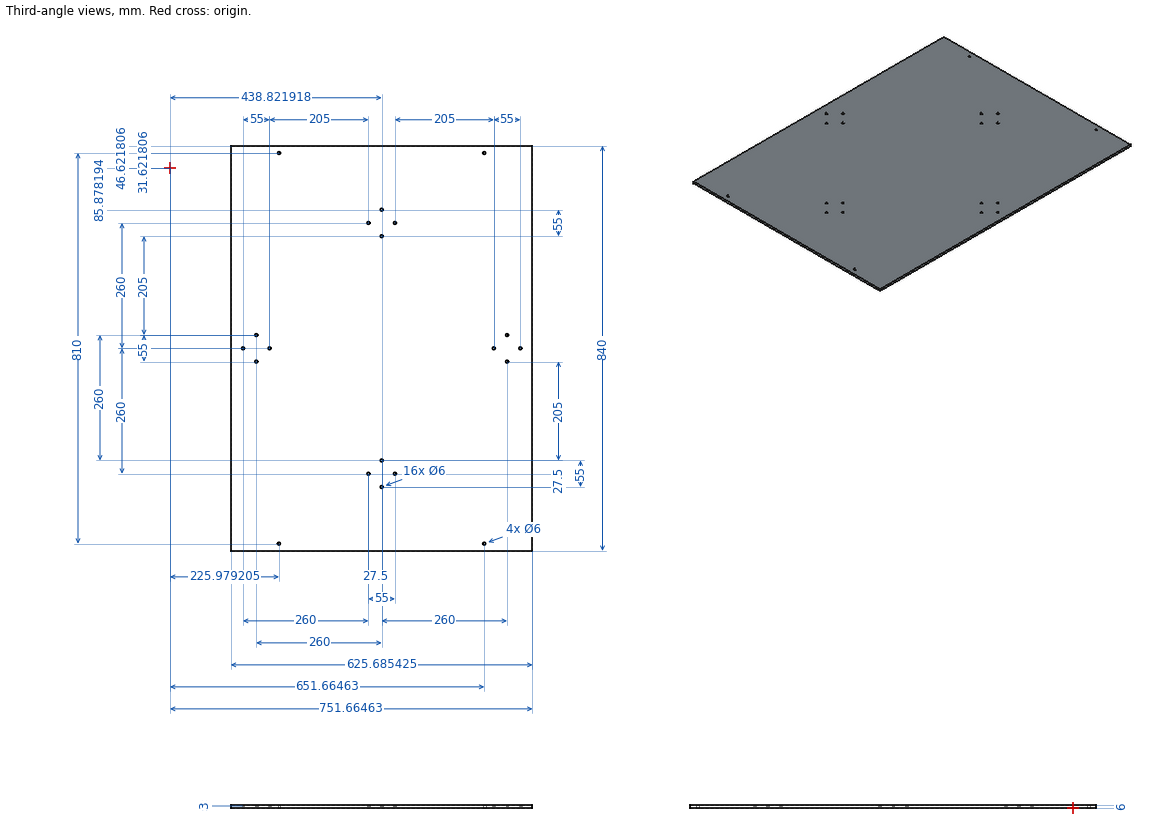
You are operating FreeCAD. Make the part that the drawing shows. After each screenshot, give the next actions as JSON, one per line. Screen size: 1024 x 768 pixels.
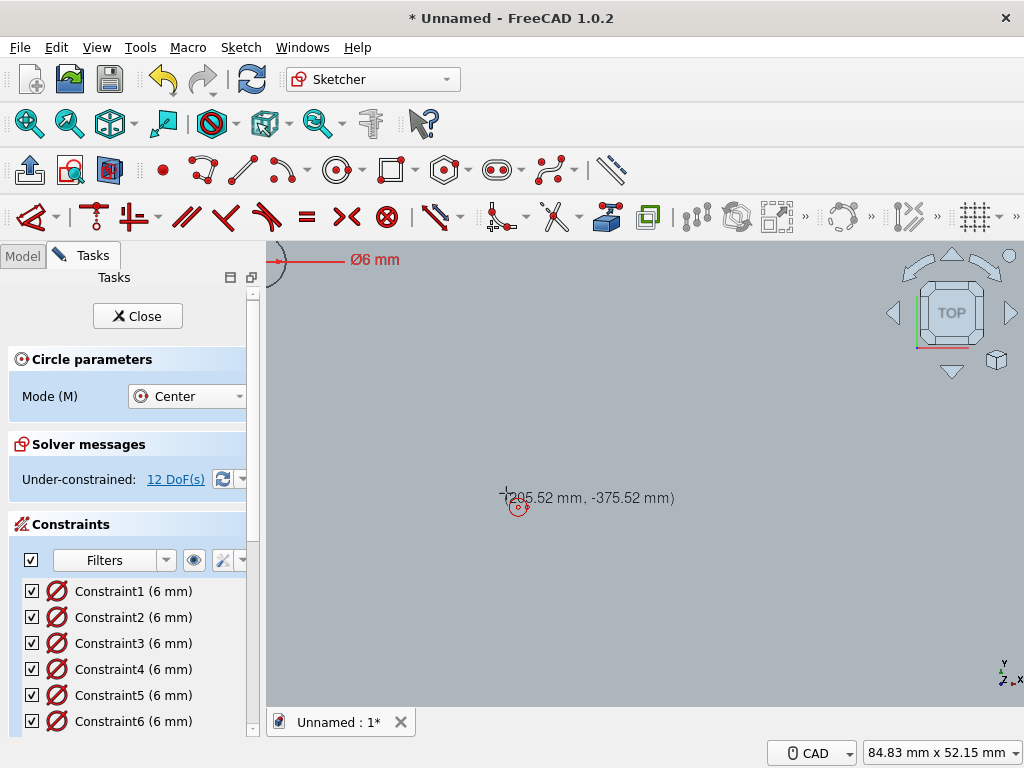
{"action": "scroll", "coordinate": [506, 493], "scroll_direction": "down", "scroll_amount": 15}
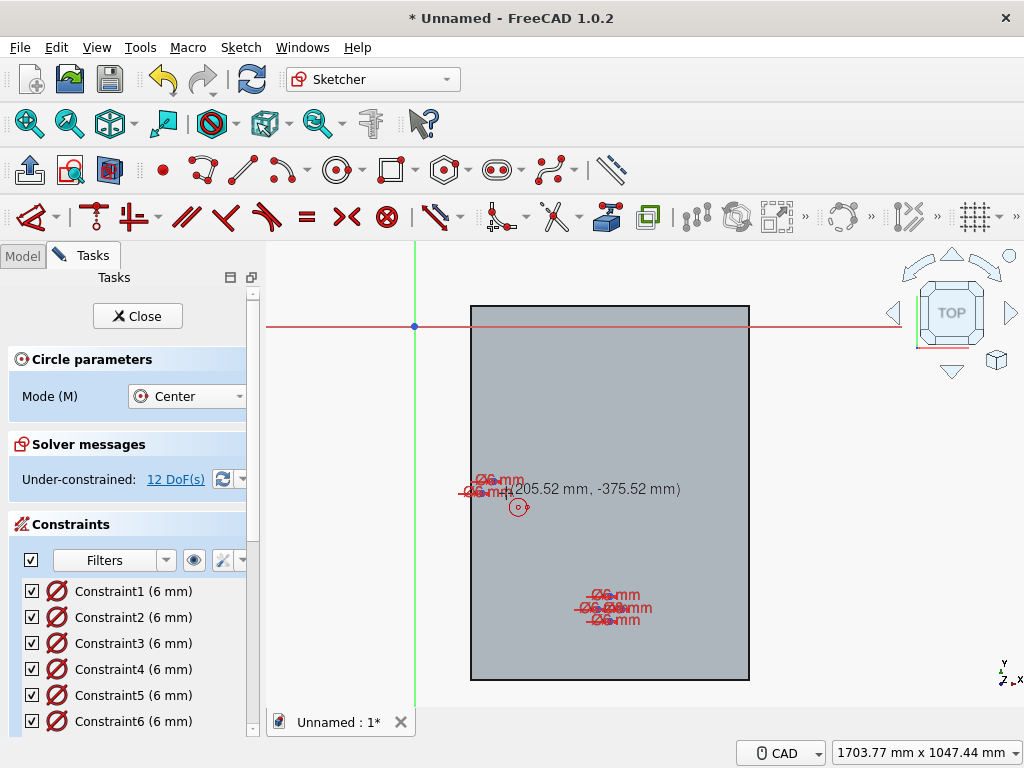
{"action": "left_click", "coordinate": [506, 493]}
{"action": "mouse_move", "coordinate": [507, 492]}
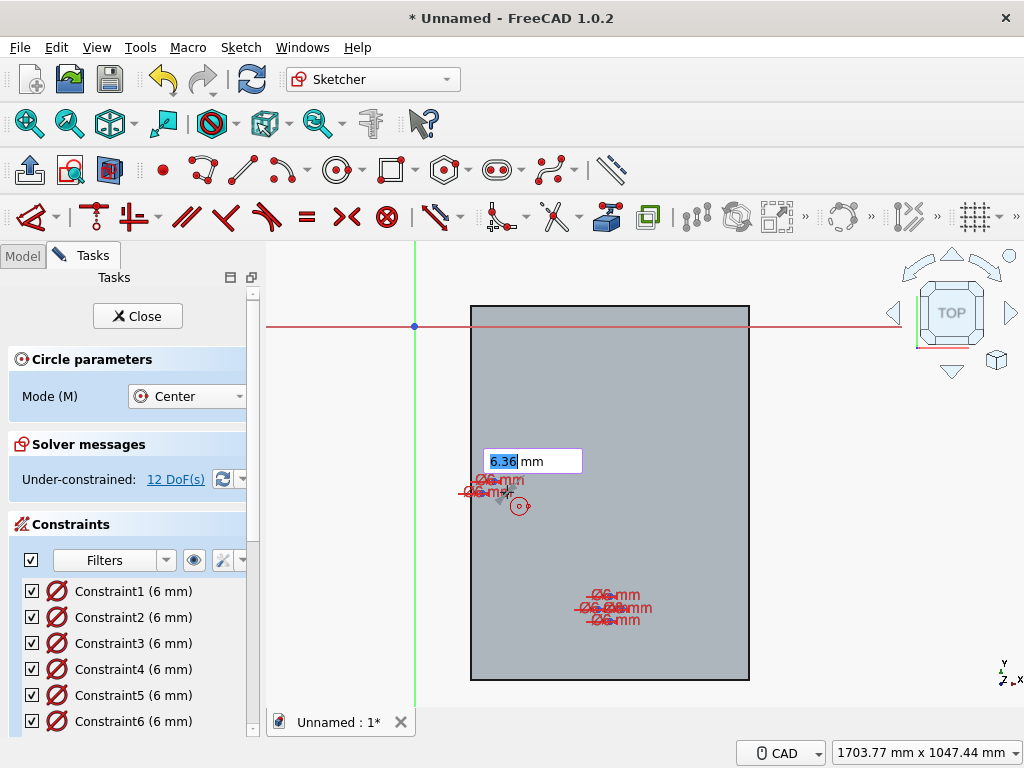
{"action": "type", "text": "6"}
{"action": "key", "text": "Return"}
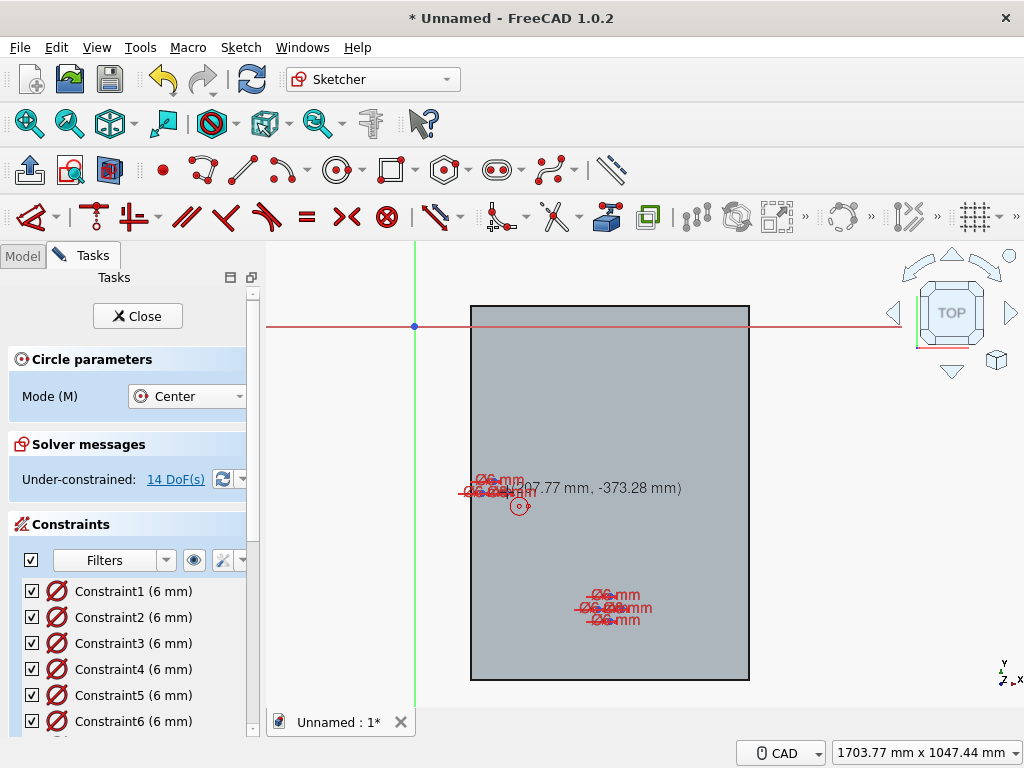
{"action": "scroll", "coordinate": [494, 505], "scroll_direction": "up", "scroll_amount": 15}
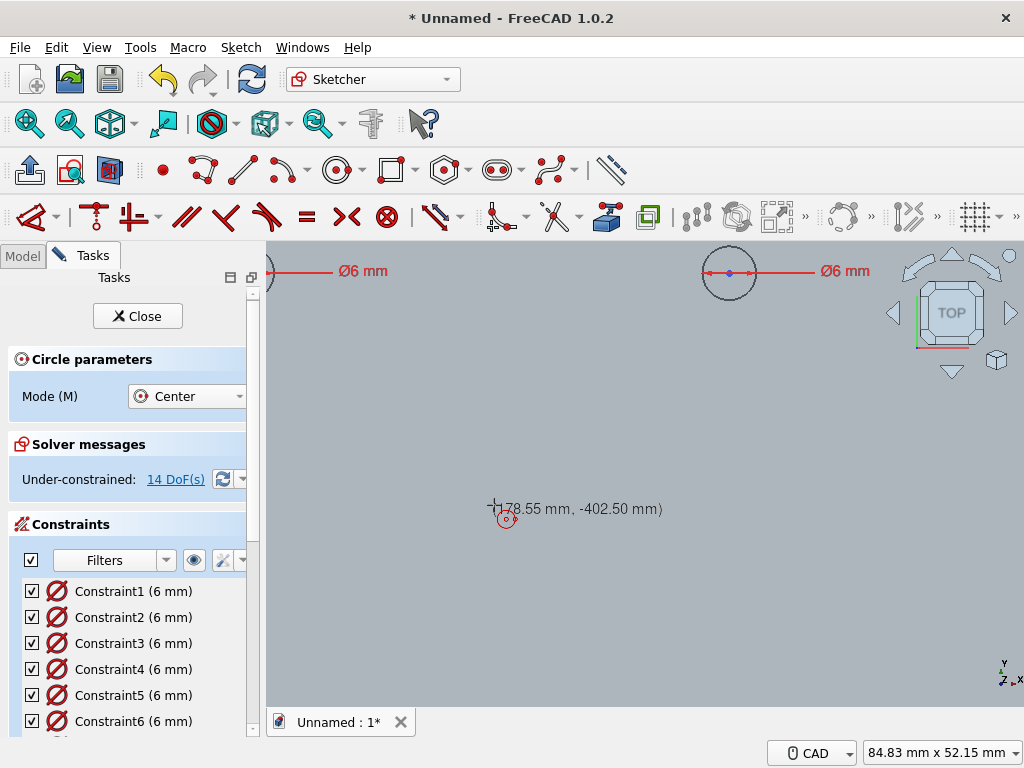
{"action": "scroll", "coordinate": [494, 505], "scroll_direction": "down", "scroll_amount": 15}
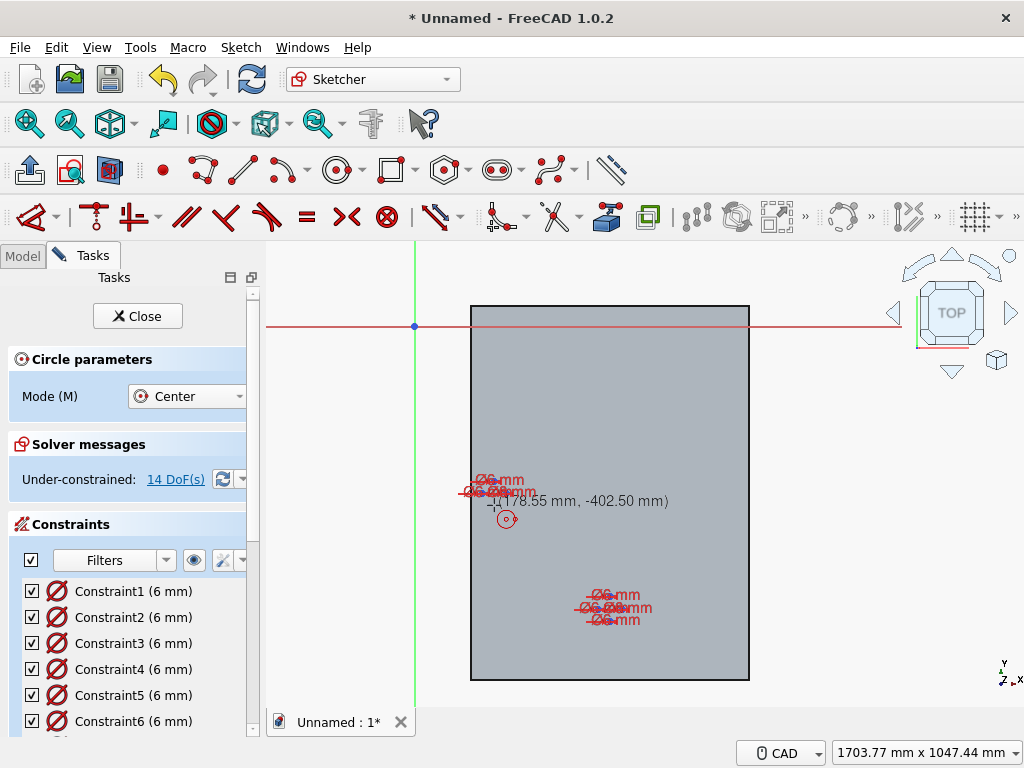
{"action": "left_click", "coordinate": [494, 505]}
{"action": "mouse_move", "coordinate": [495, 504]}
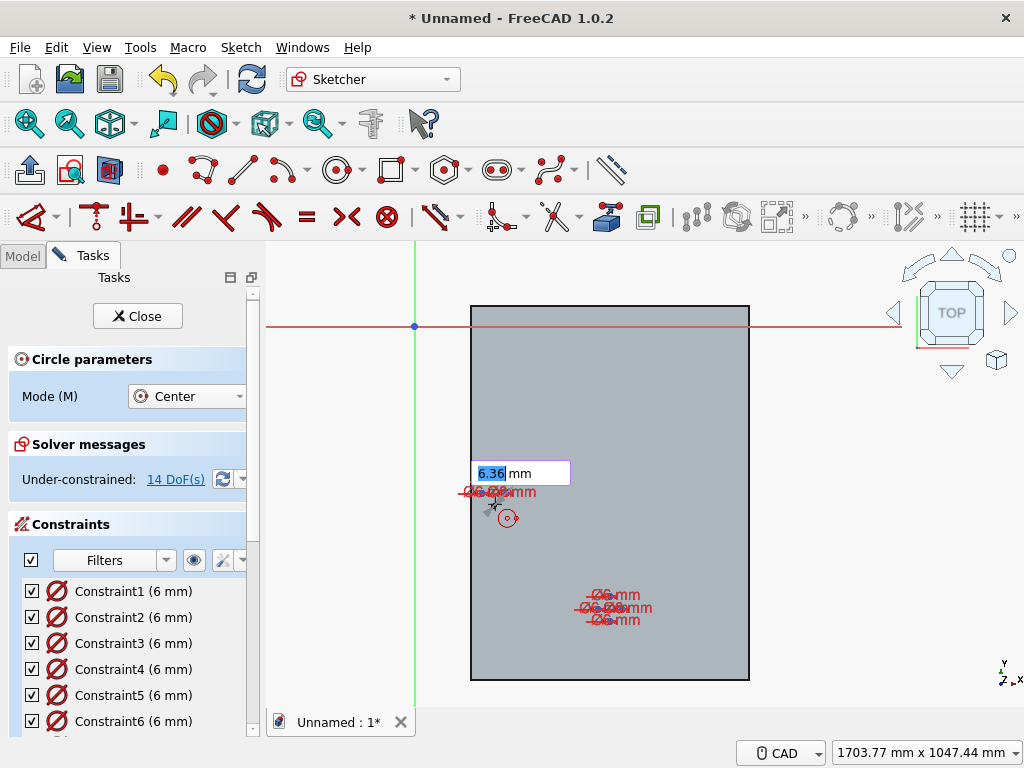
{"action": "type", "text": "6"}
{"action": "key", "text": "Return"}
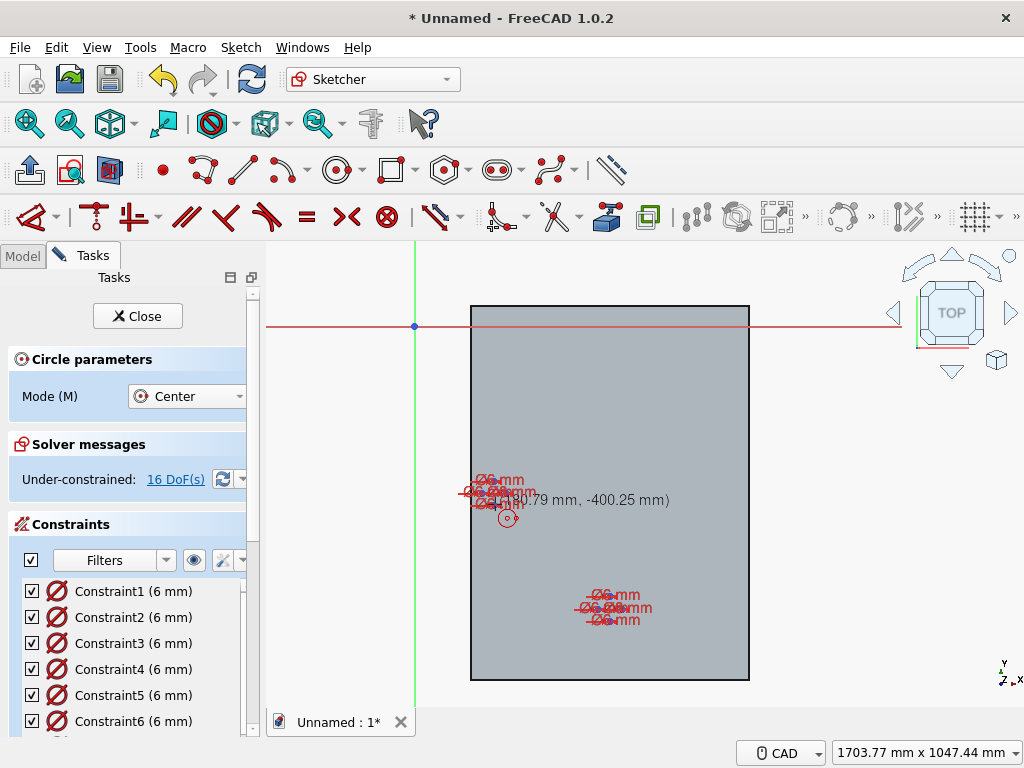
{"action": "scroll", "coordinate": [610, 390], "scroll_direction": "up", "scroll_amount": 15}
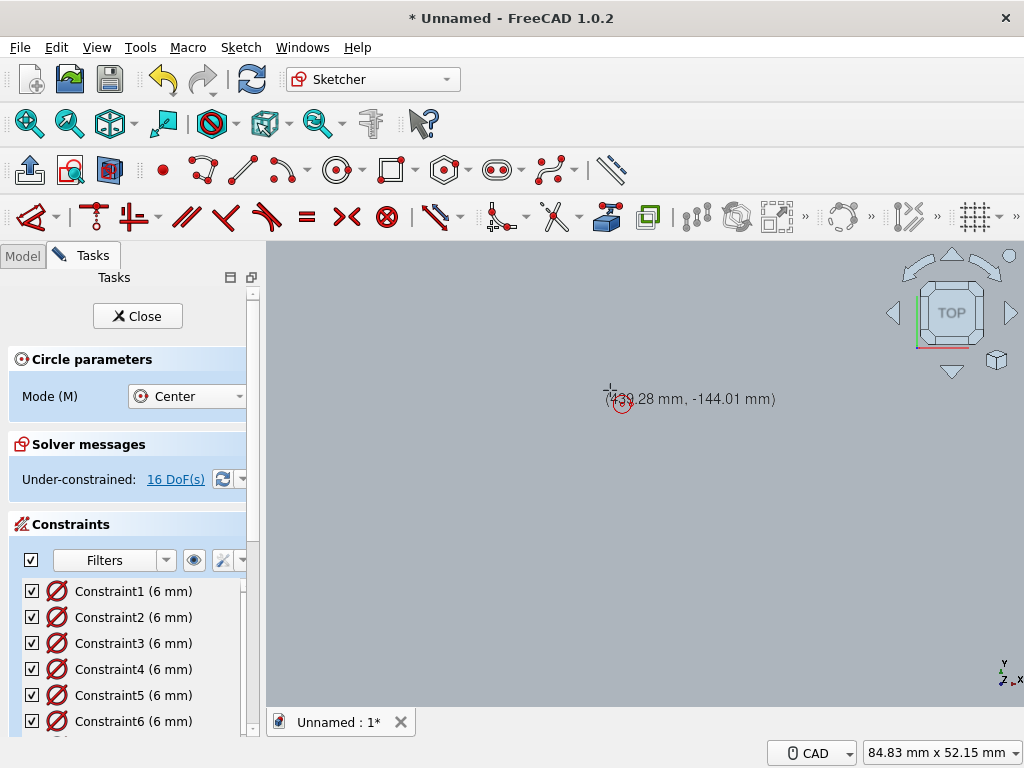
{"action": "scroll", "coordinate": [610, 390], "scroll_direction": "down", "scroll_amount": 15}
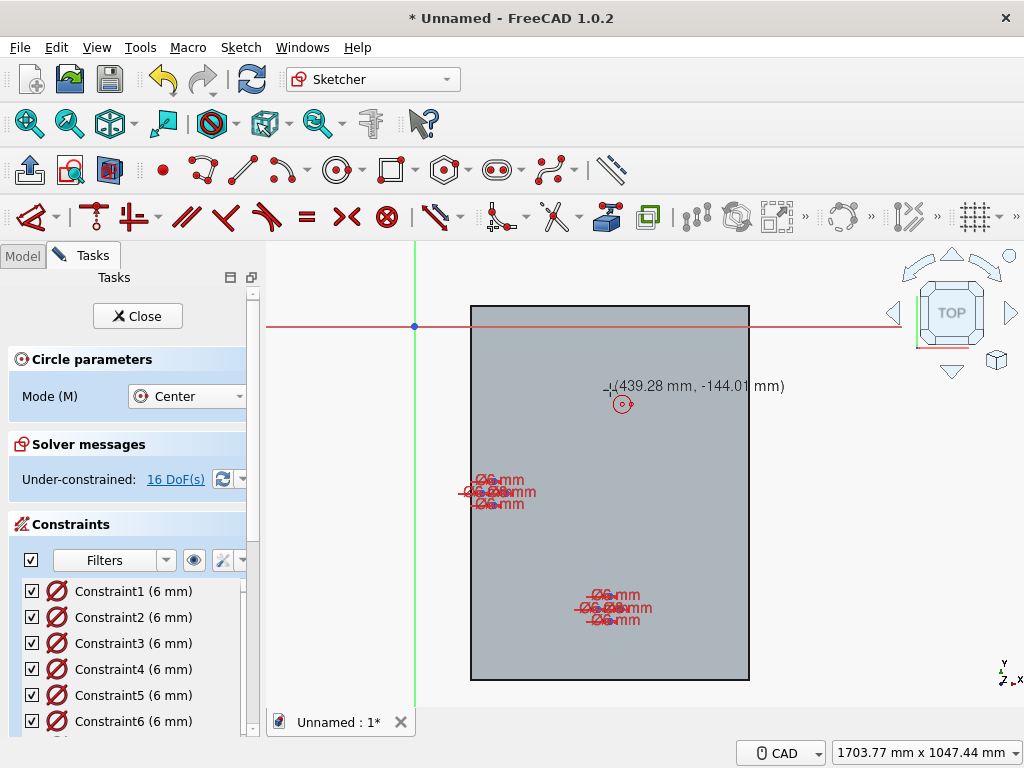
{"action": "left_click", "coordinate": [610, 390]}
{"action": "mouse_move", "coordinate": [611, 389]}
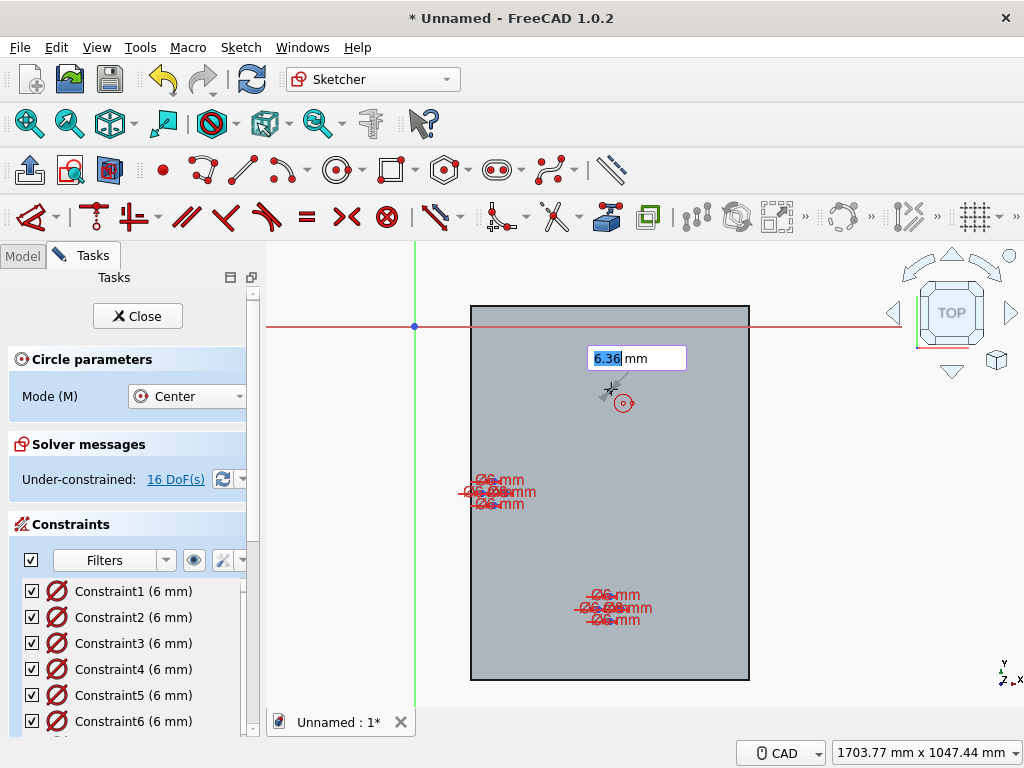
{"action": "type", "text": "6"}
{"action": "key", "text": "Return"}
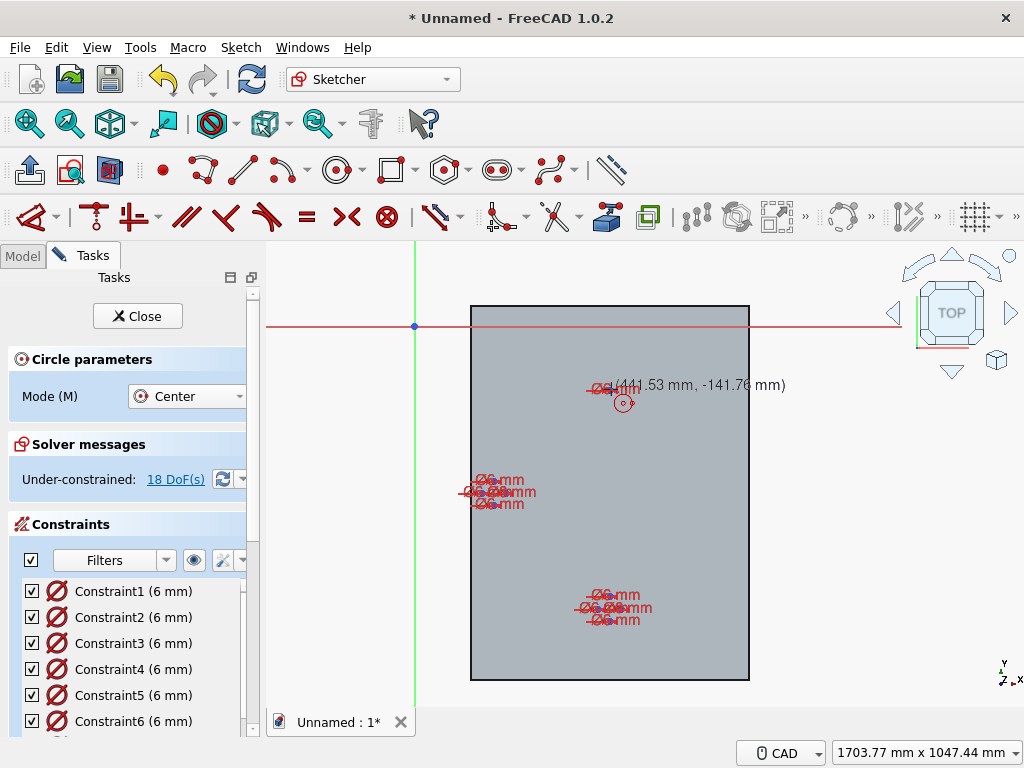
{"action": "scroll", "coordinate": [598, 377], "scroll_direction": "up", "scroll_amount": 15}